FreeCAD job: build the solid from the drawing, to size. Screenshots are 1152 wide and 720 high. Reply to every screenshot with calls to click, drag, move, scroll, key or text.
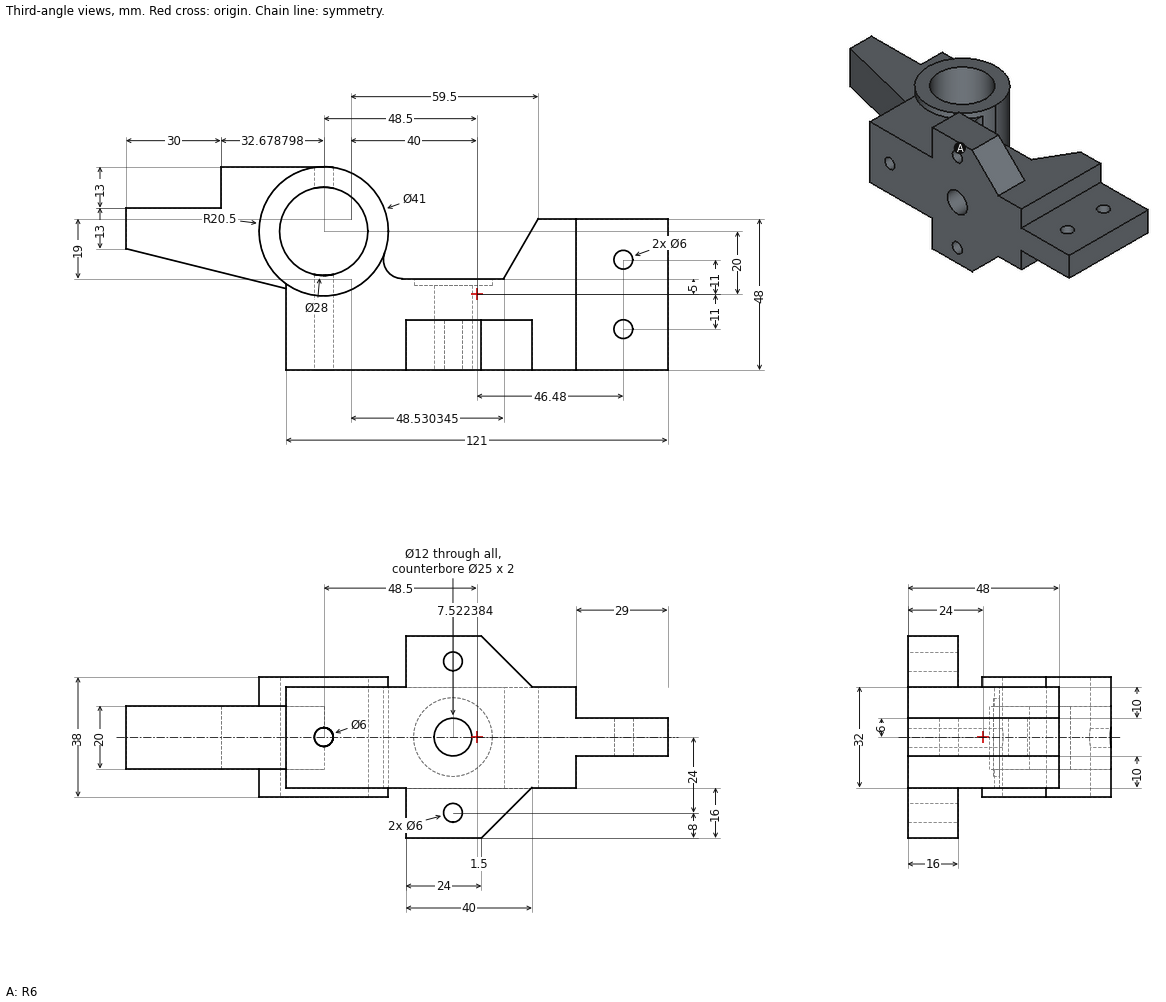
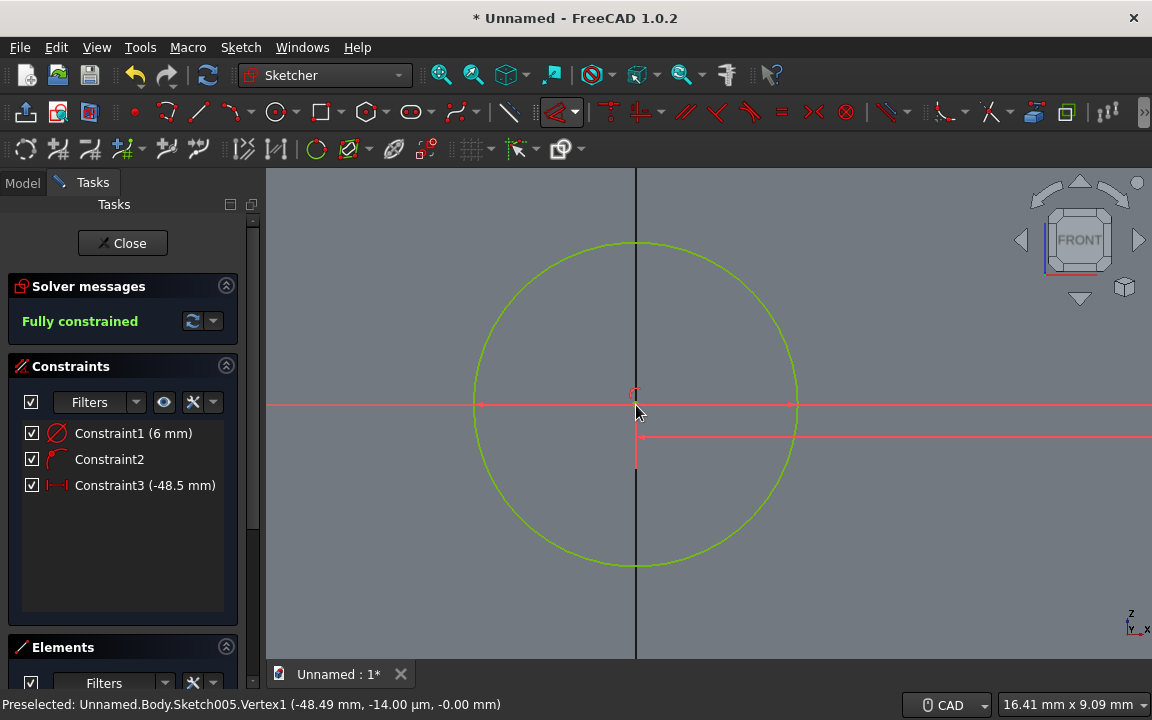
click(123, 243)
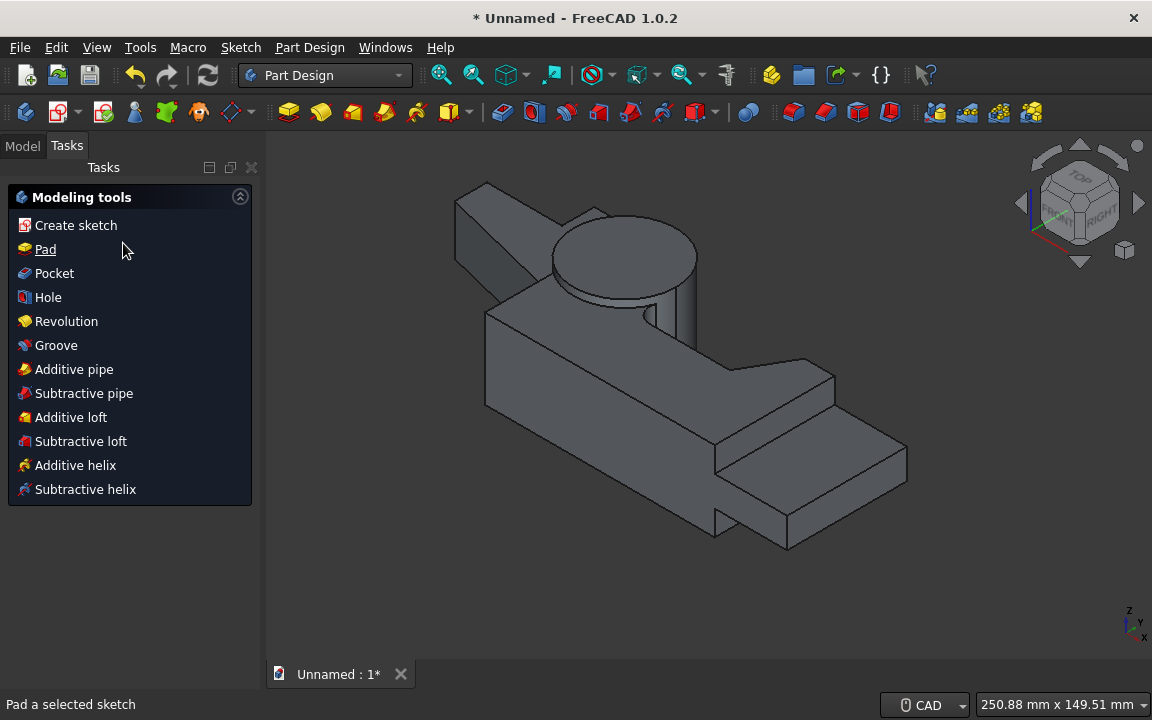
click(504, 112)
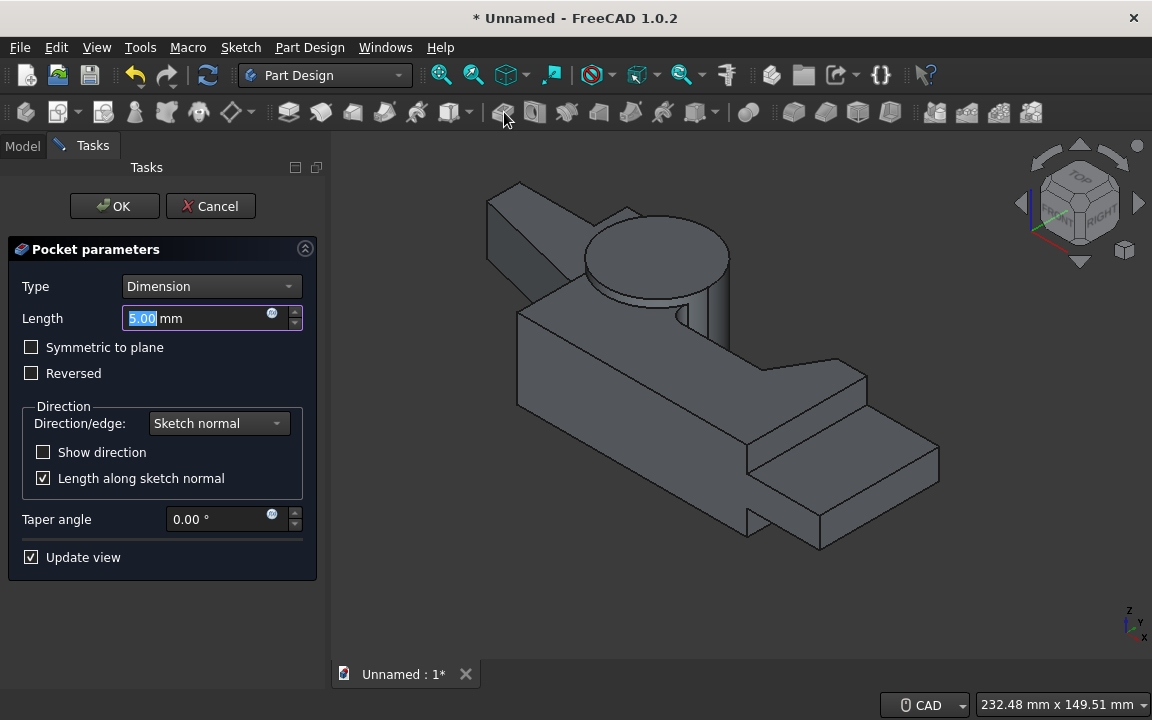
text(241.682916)
key(Tab)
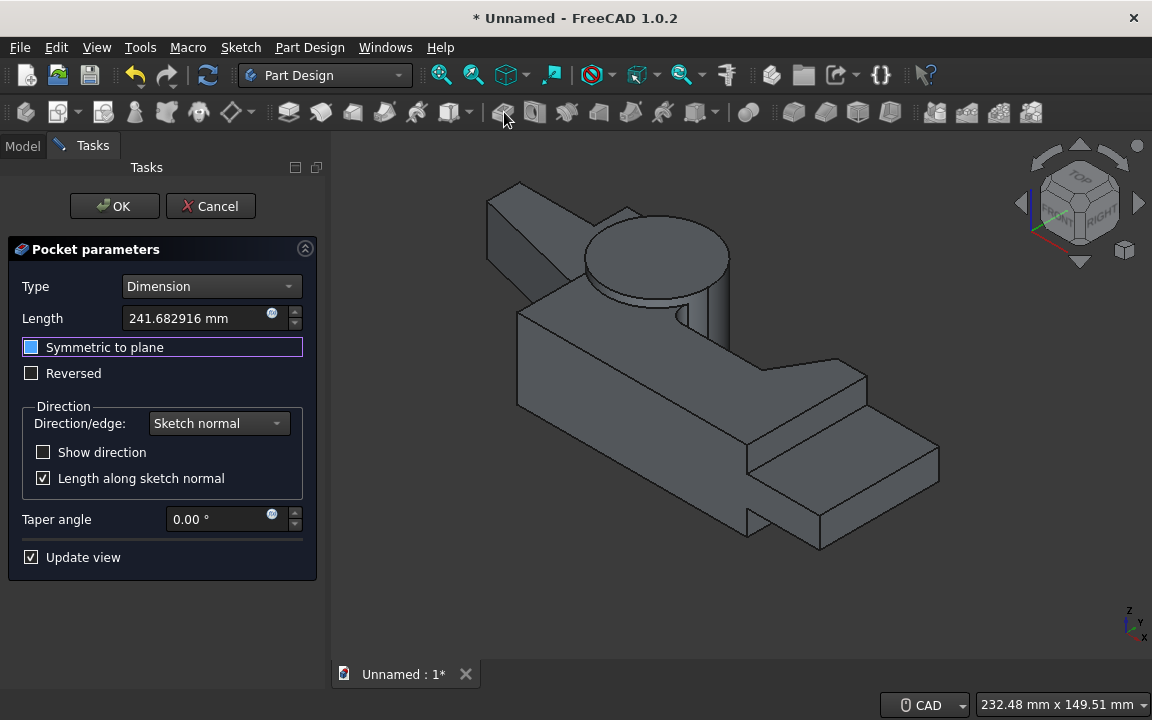
click(30, 347)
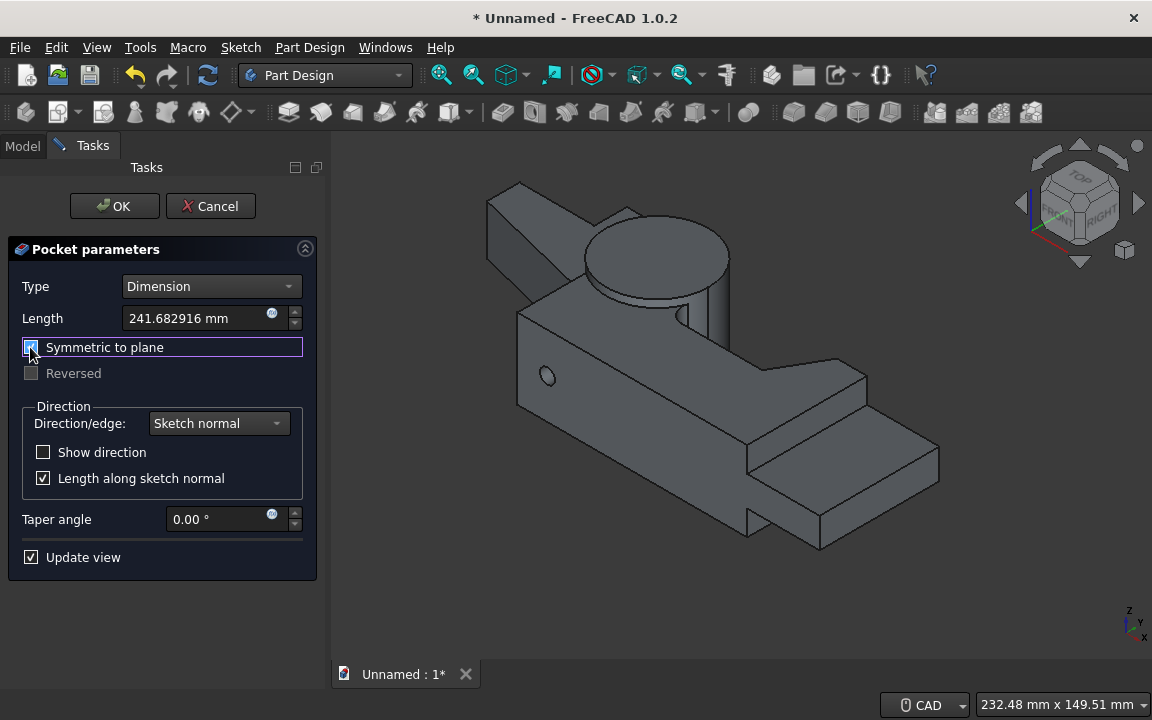
click(115, 206)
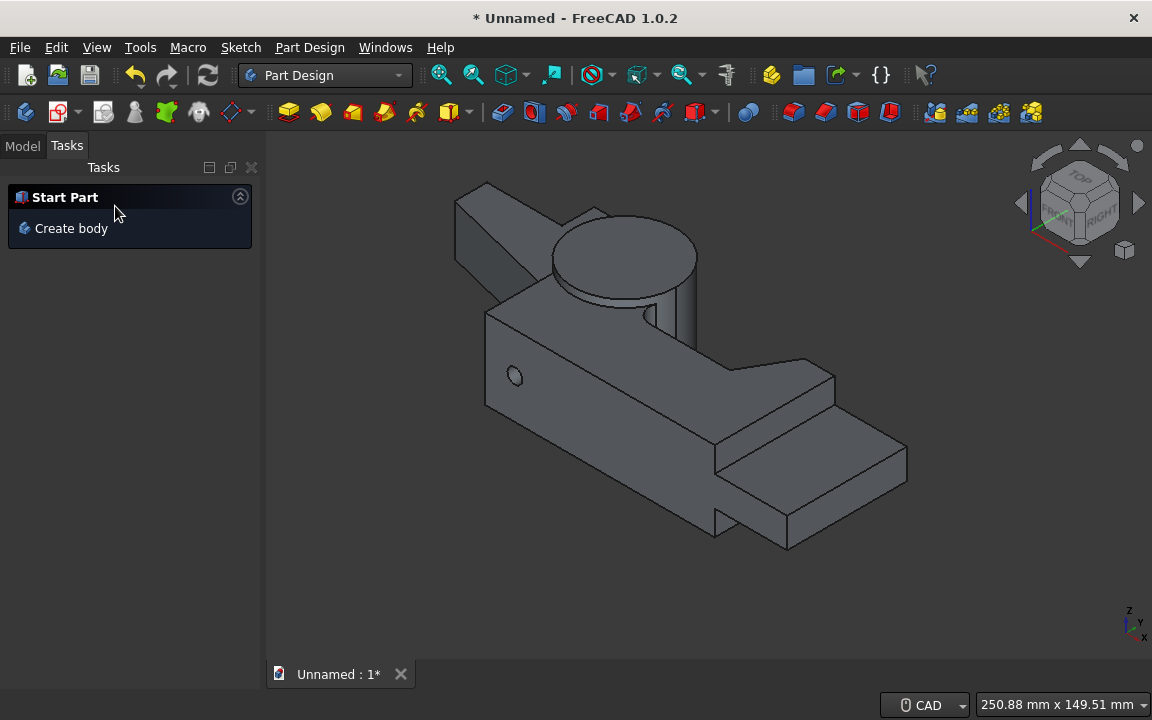
click(625, 257)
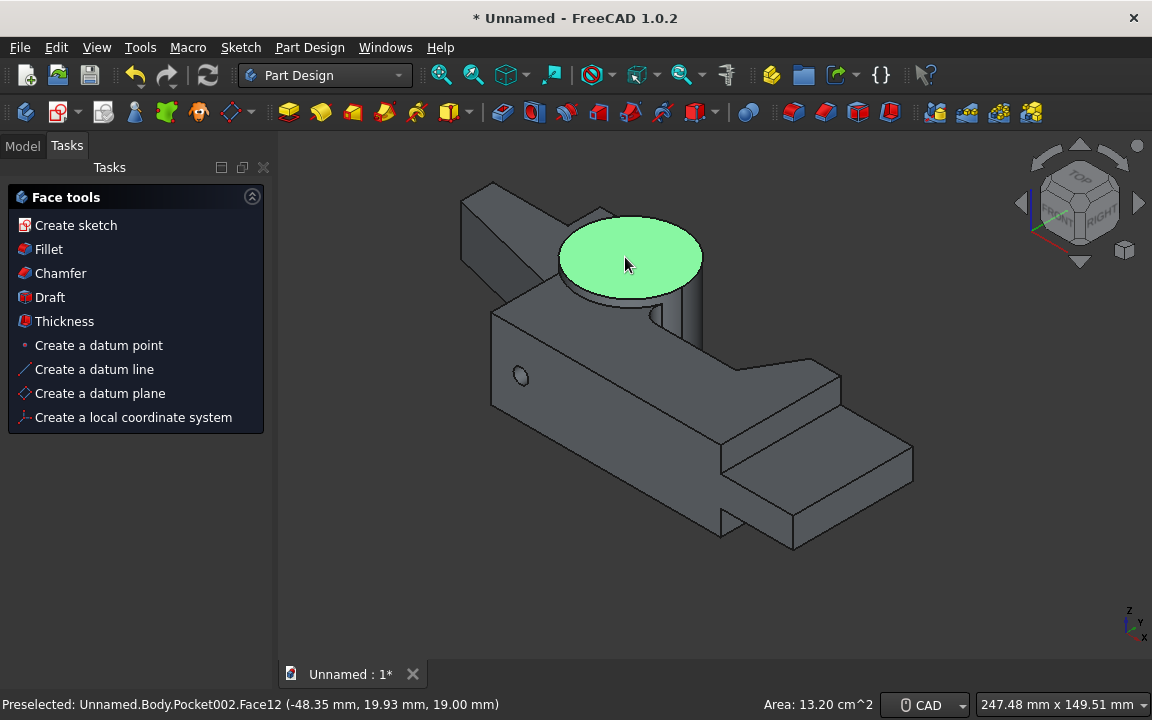
click(58, 112)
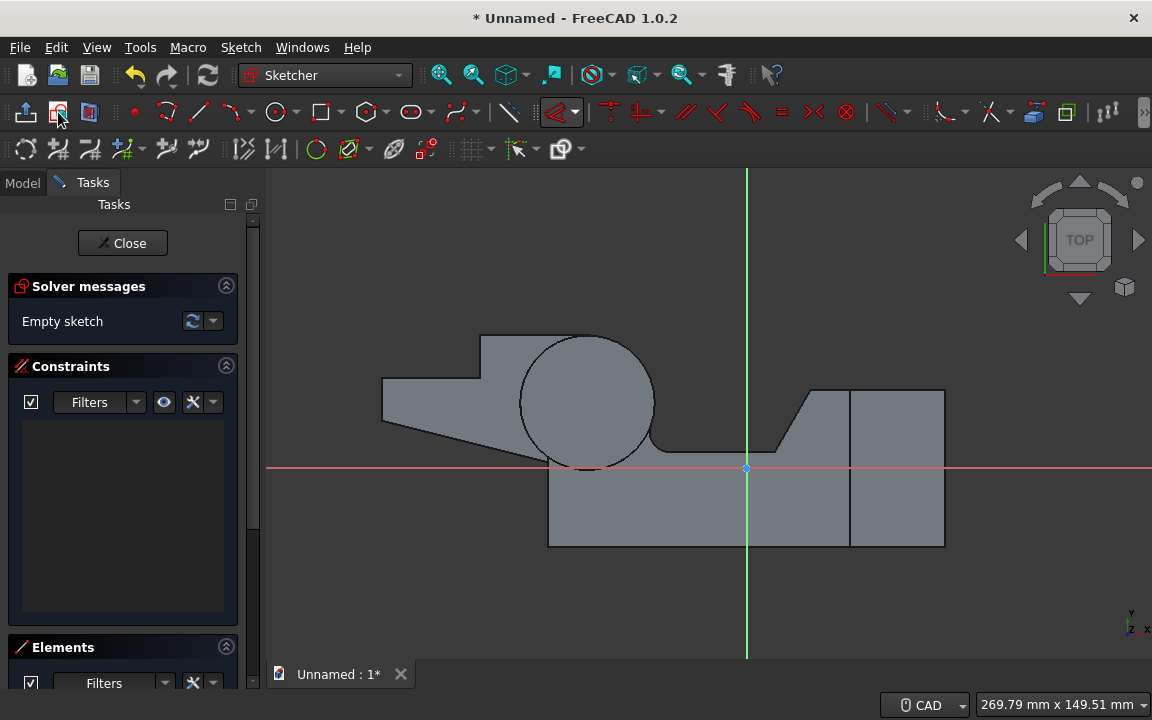
scroll(647, 412, up, 4)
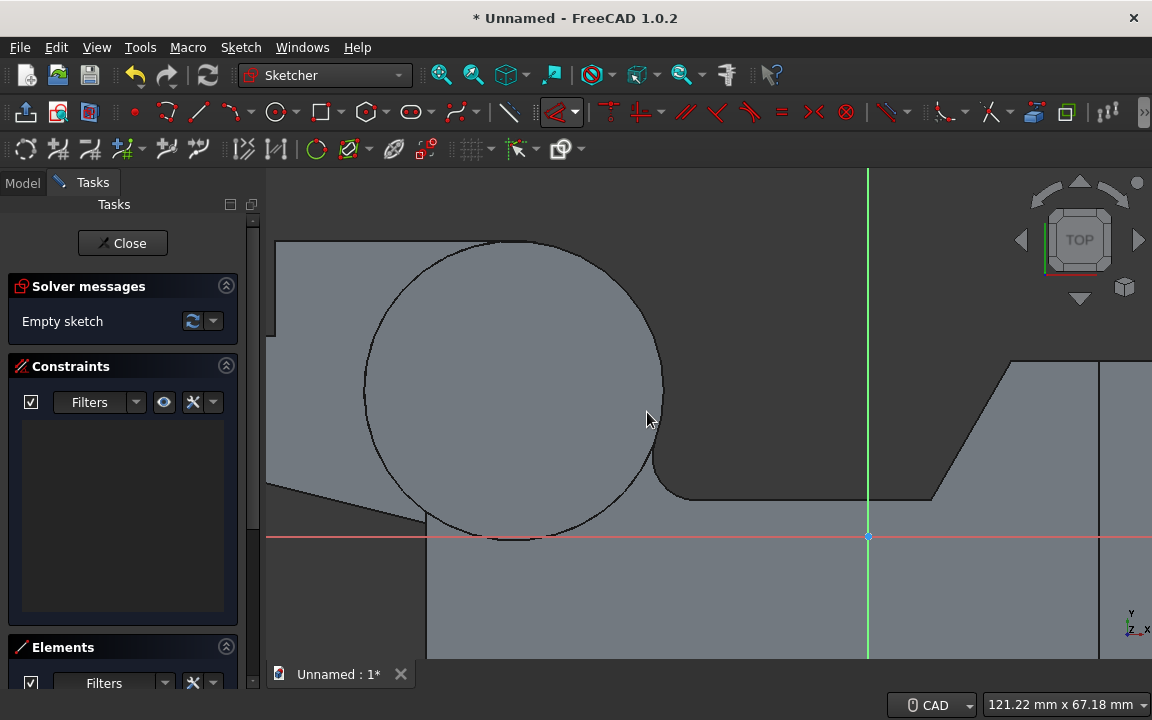
key(g)
key(c)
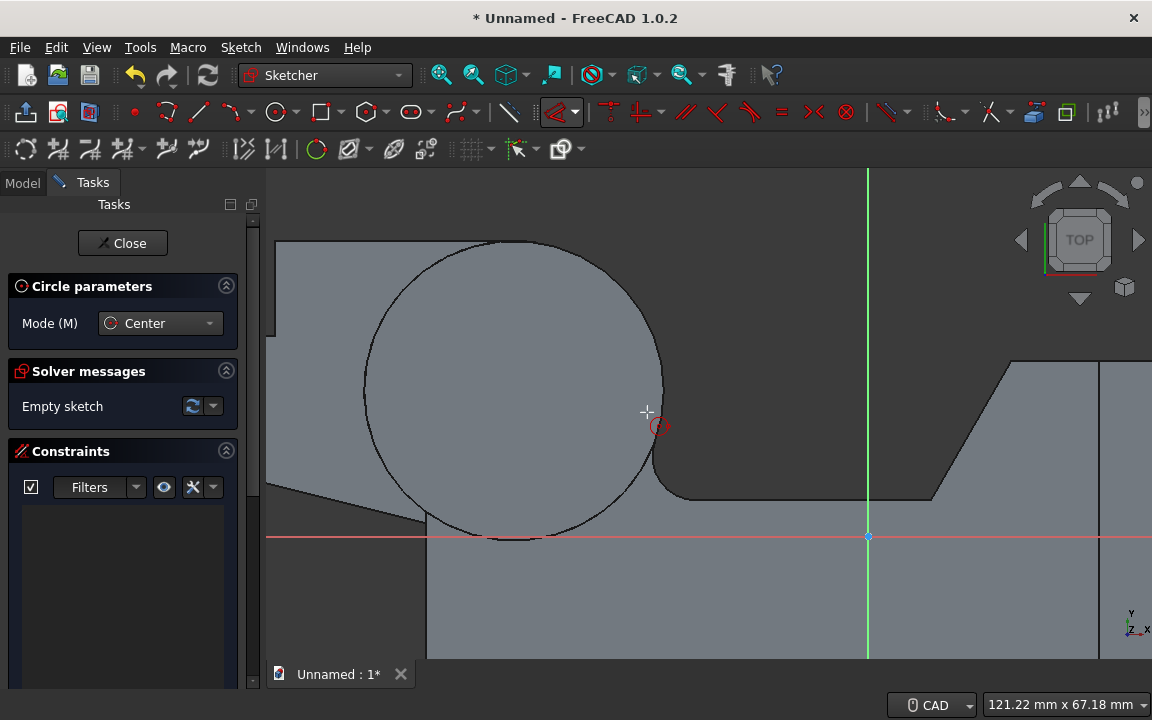
click(514, 391)
move(586, 318)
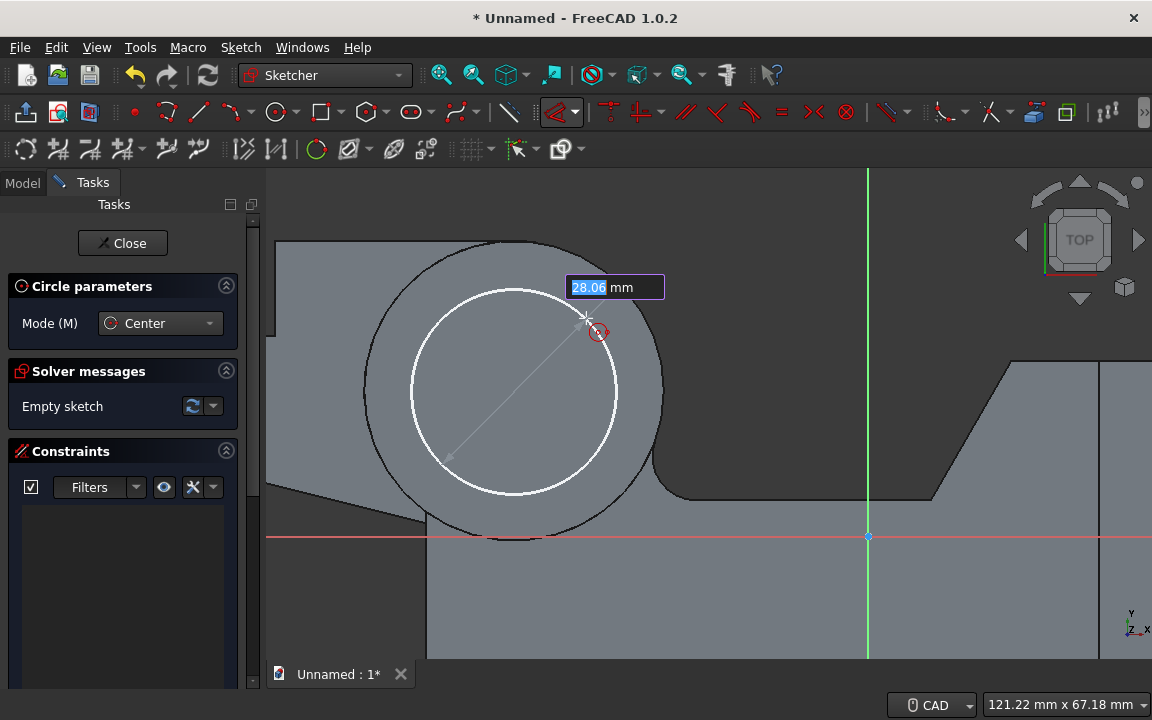
text(28)
key(Return)
key(Escape)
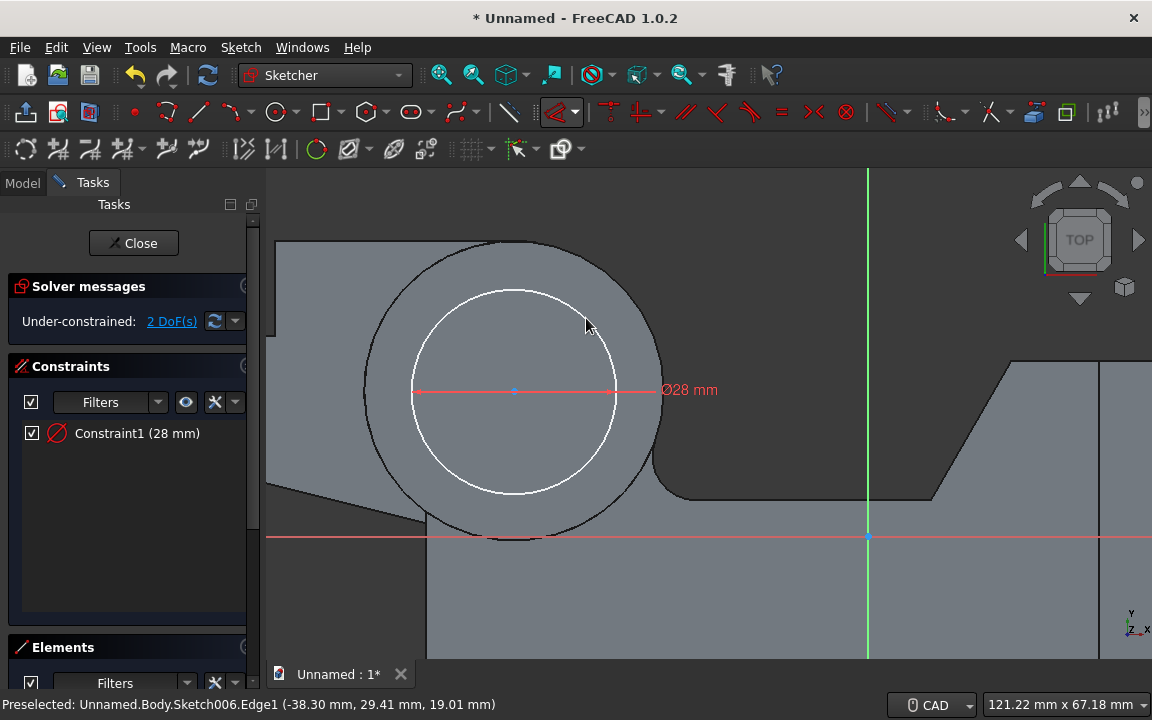
click(514, 392)